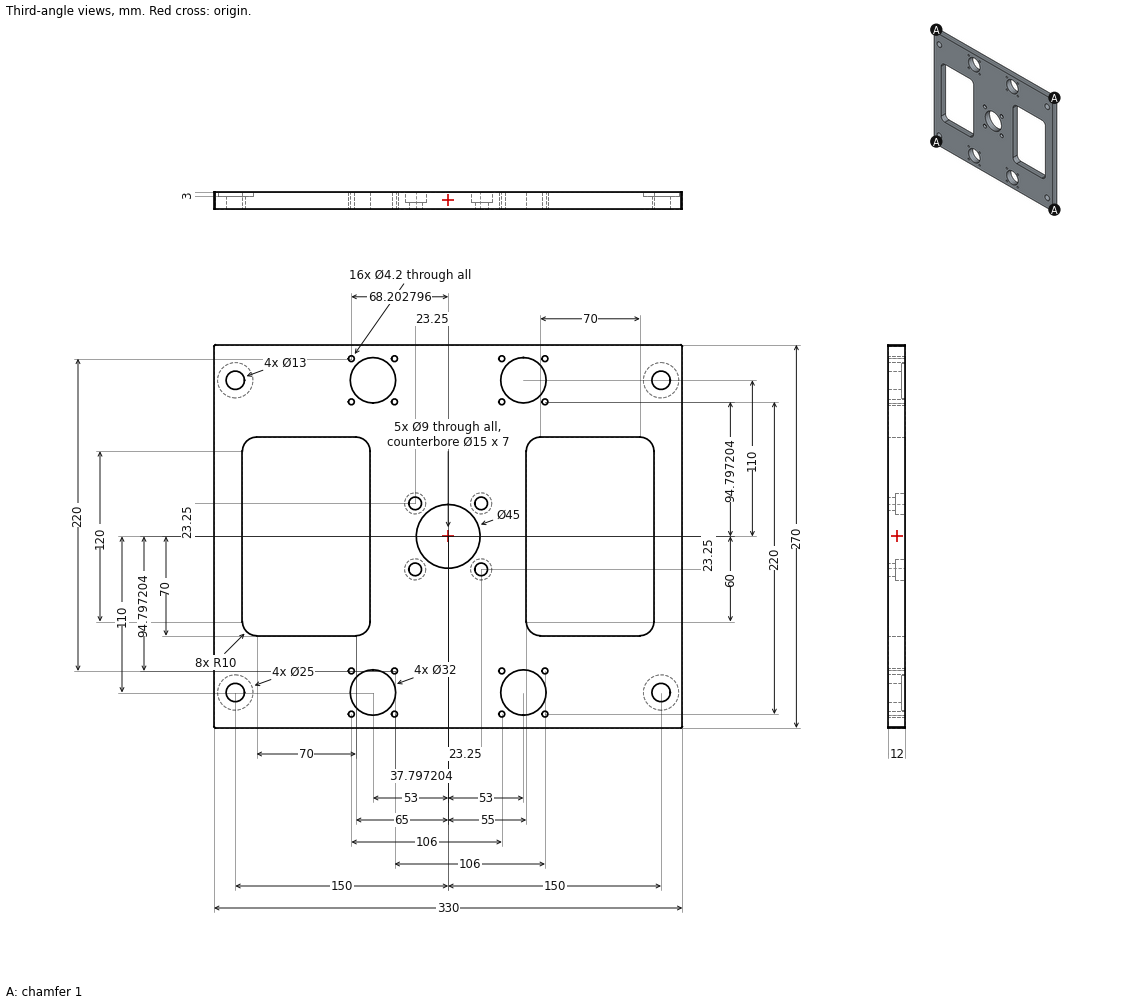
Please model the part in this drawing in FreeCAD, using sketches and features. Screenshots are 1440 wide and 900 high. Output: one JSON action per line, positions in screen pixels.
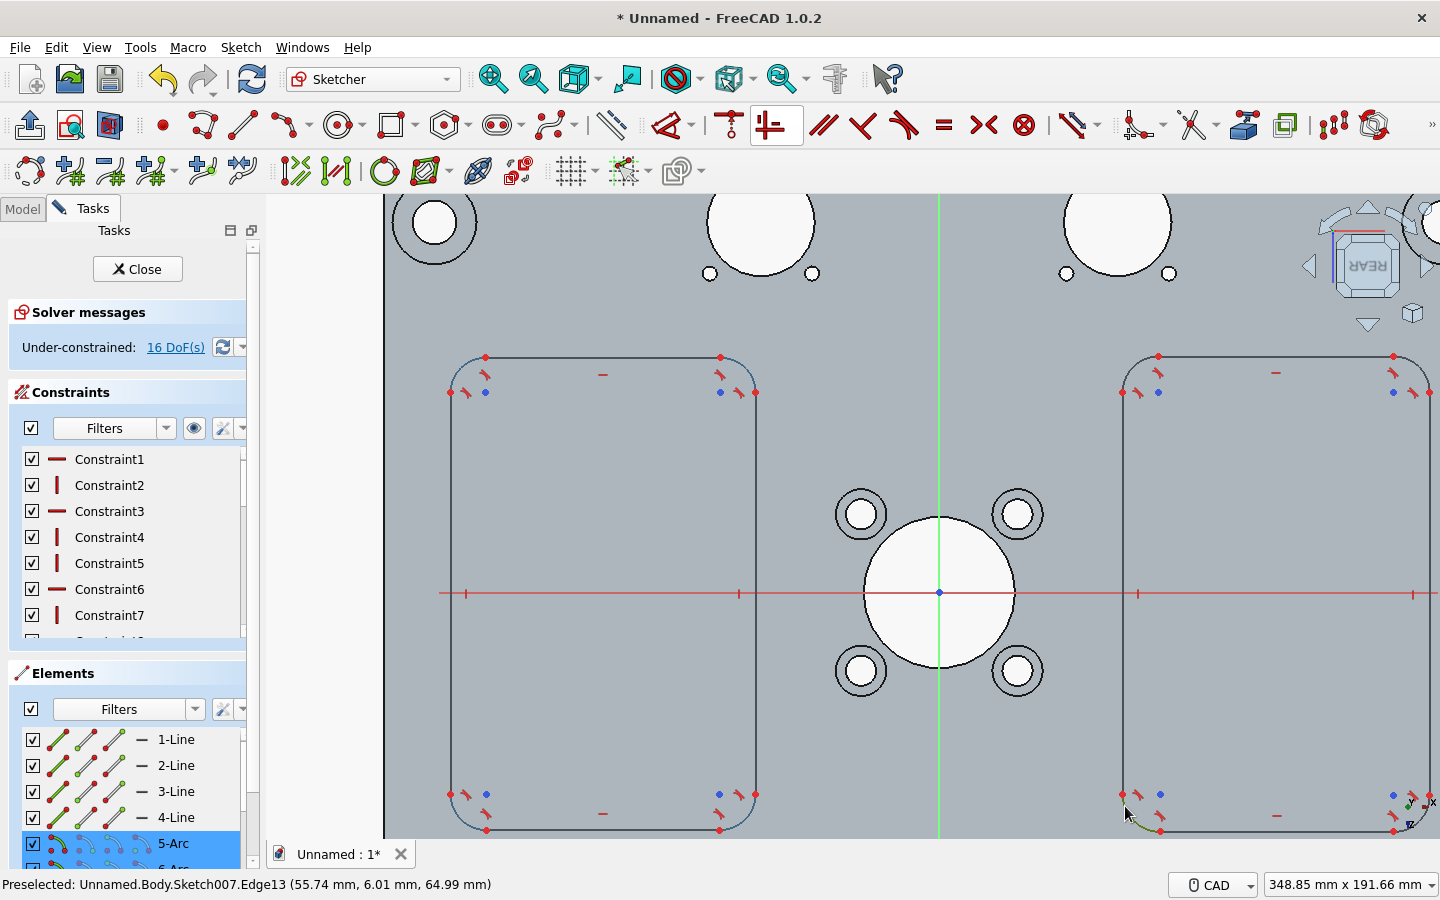
{"action": "scroll", "coordinate": [470, 362], "scroll_direction": "down", "scroll_amount": 2}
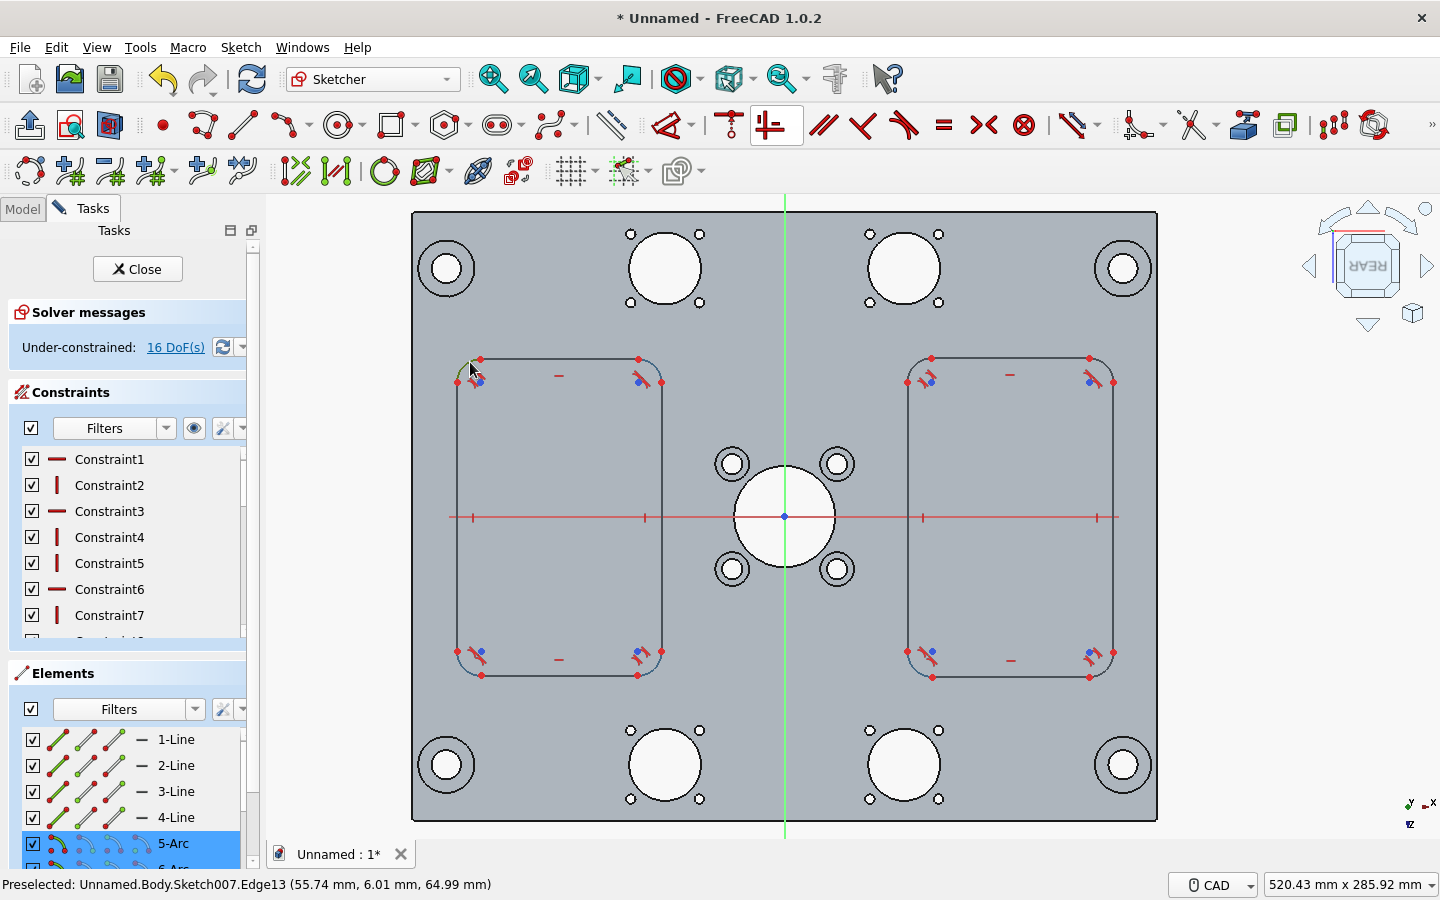
{"action": "scroll", "coordinate": [1100, 674], "scroll_direction": "up", "scroll_amount": 2}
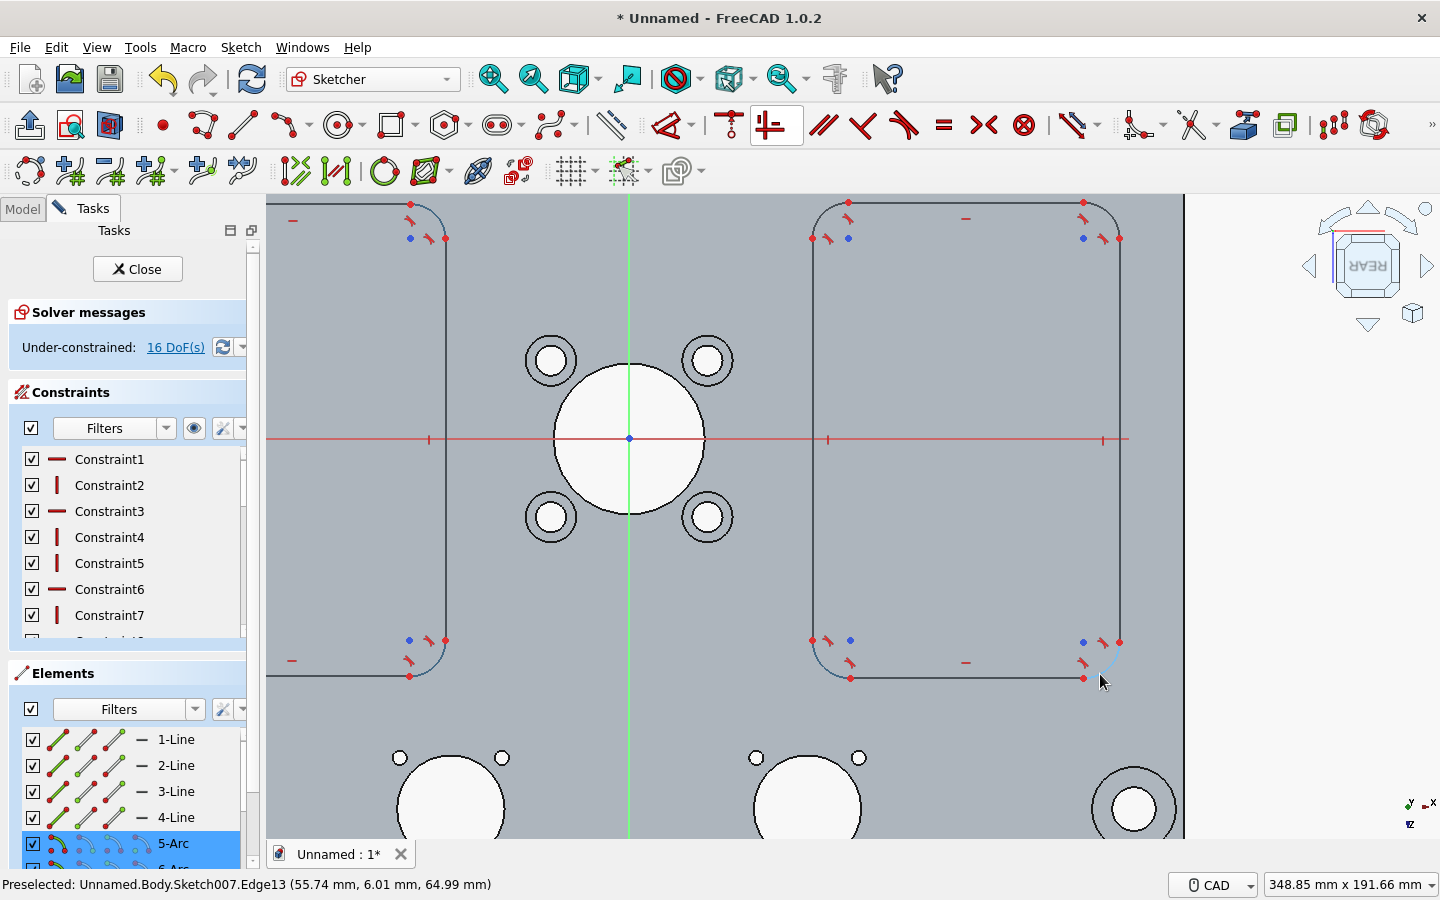
{"action": "left_click", "coordinate": [1100, 674]}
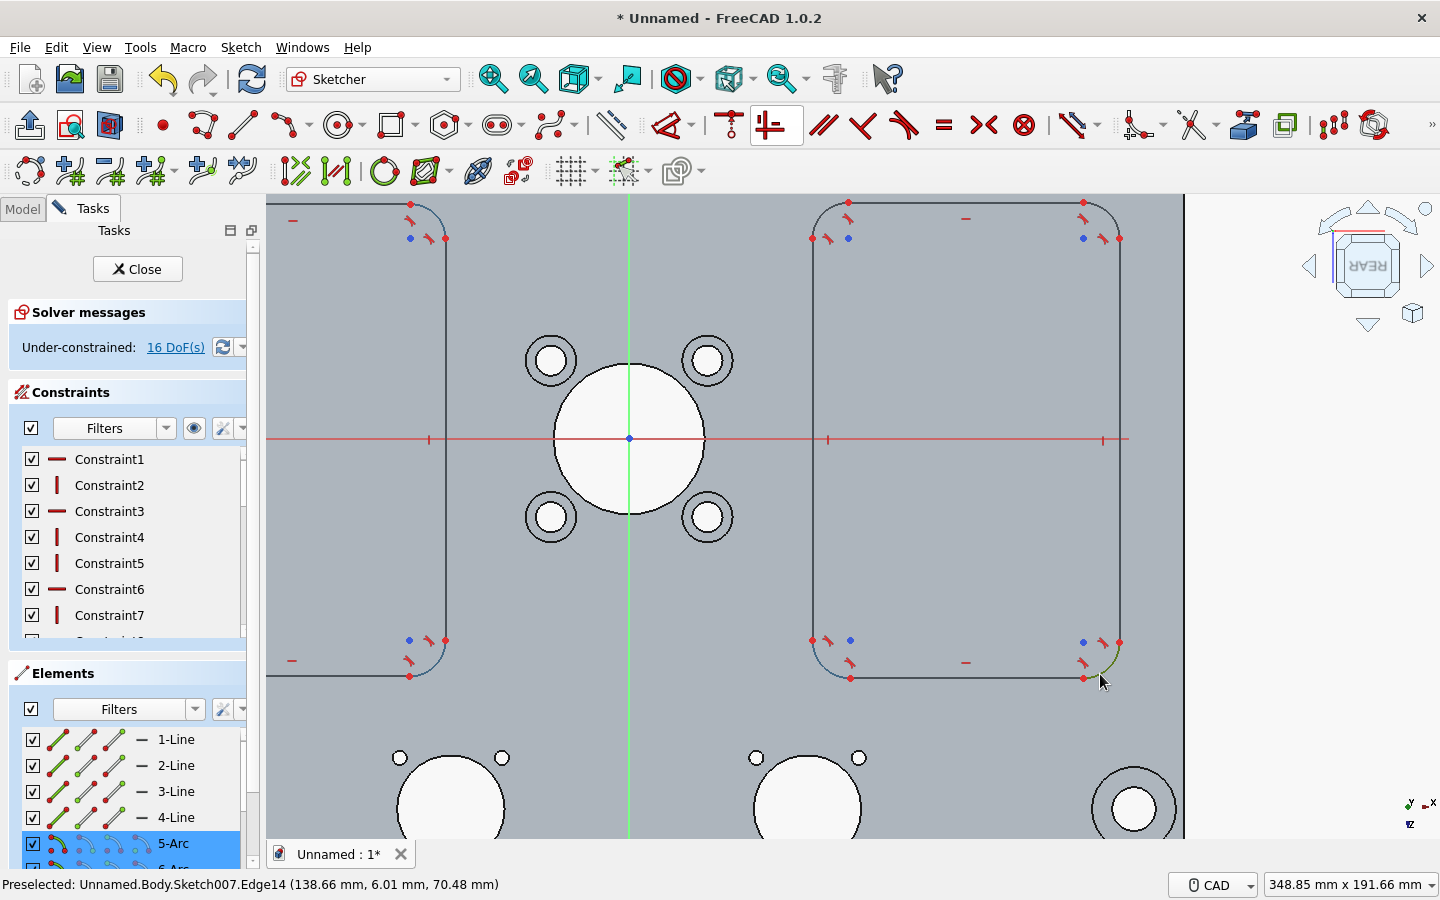
{"action": "left_click", "coordinate": [1116, 222]}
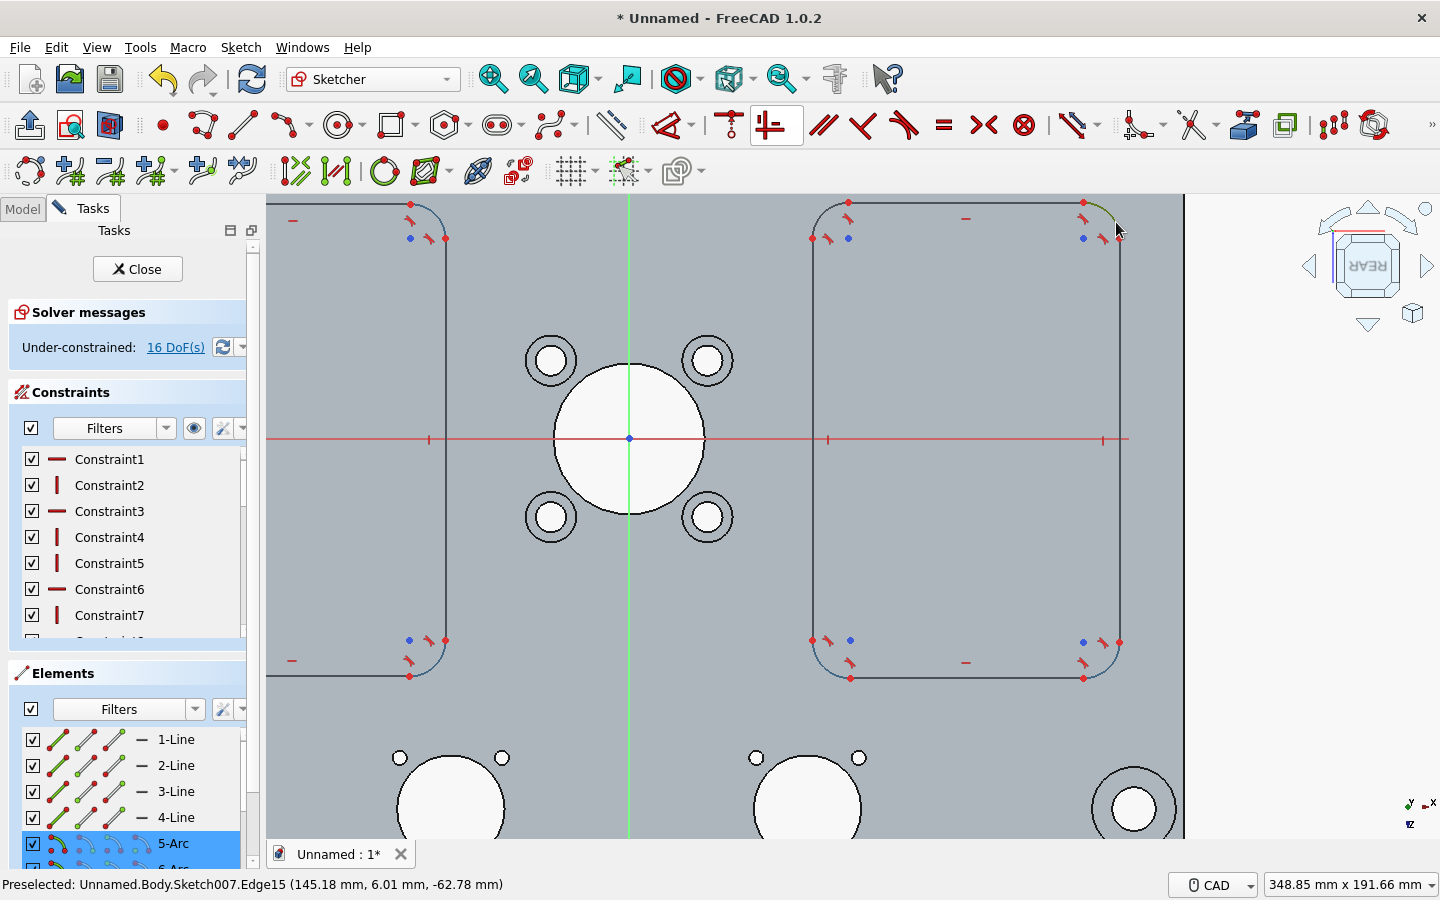
{"action": "left_click", "coordinate": [817, 222]}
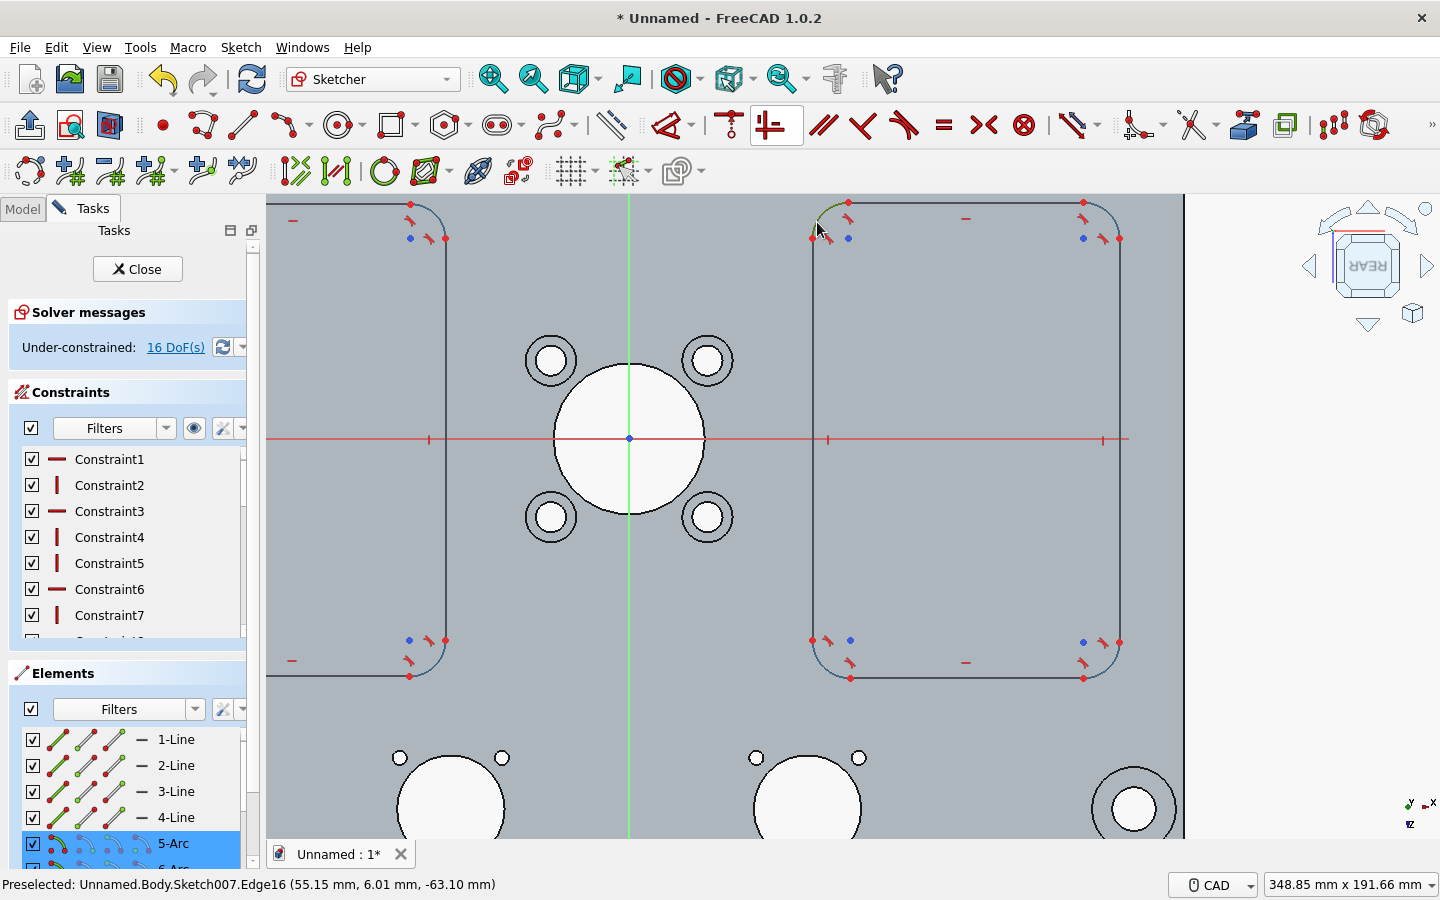
{"action": "left_click", "coordinate": [944, 126]}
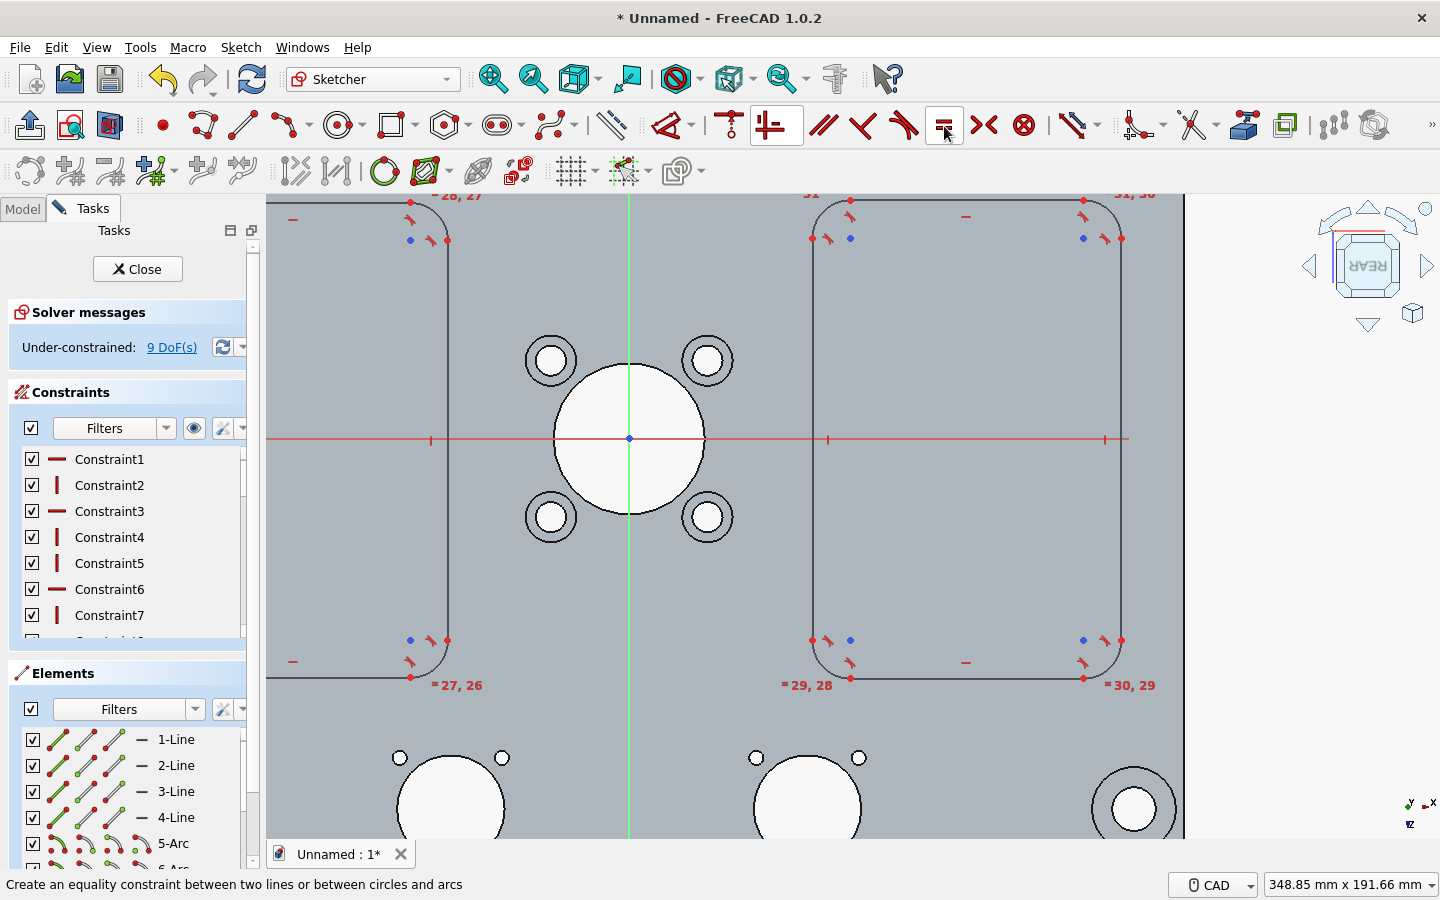
{"action": "key", "text": "d"}